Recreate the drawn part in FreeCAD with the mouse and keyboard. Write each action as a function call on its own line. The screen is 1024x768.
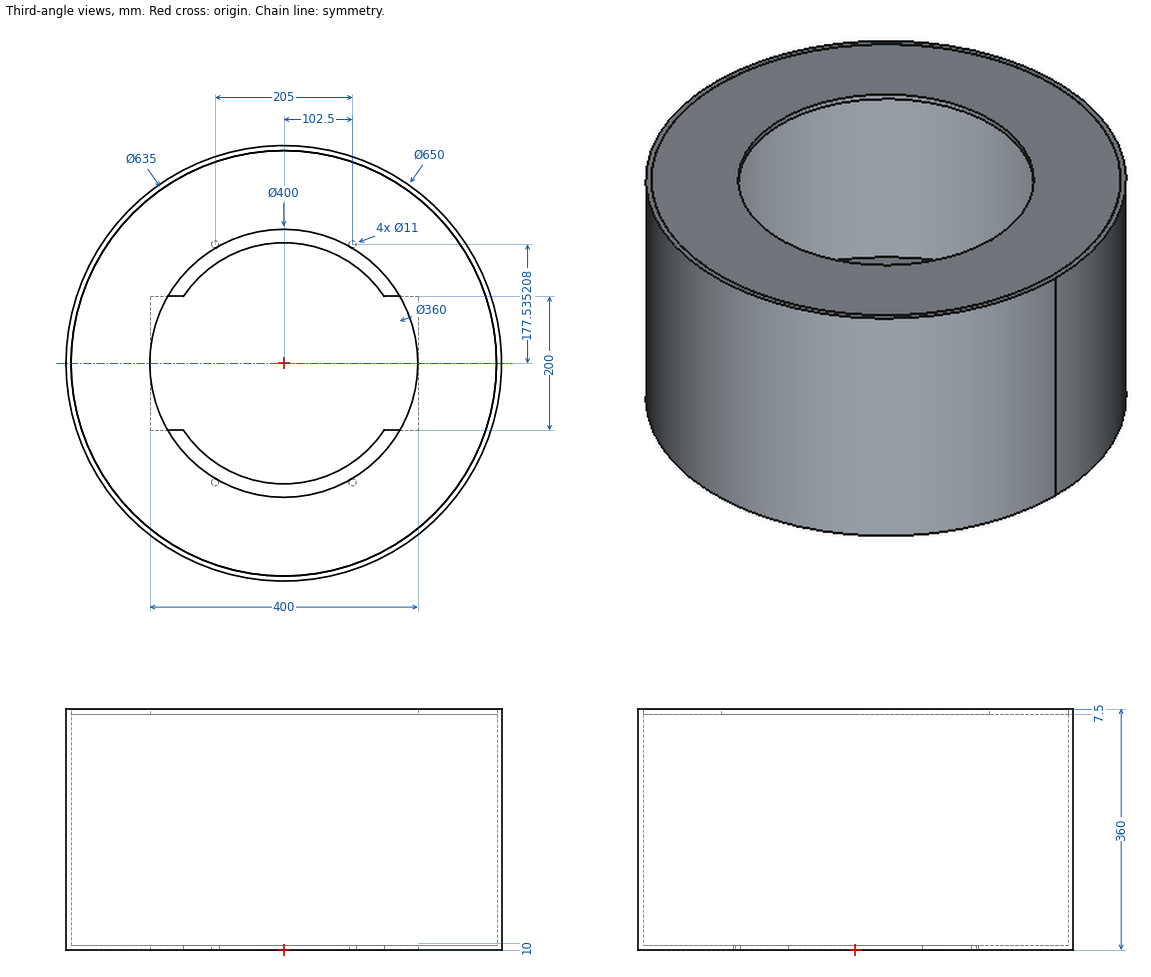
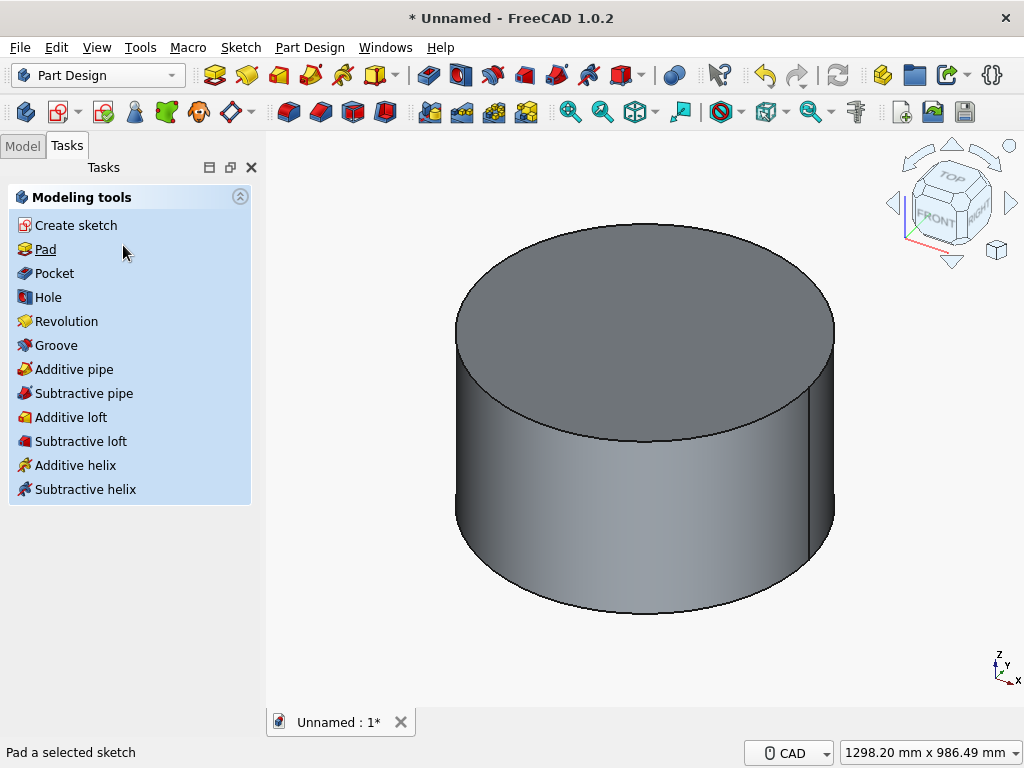
click(430, 76)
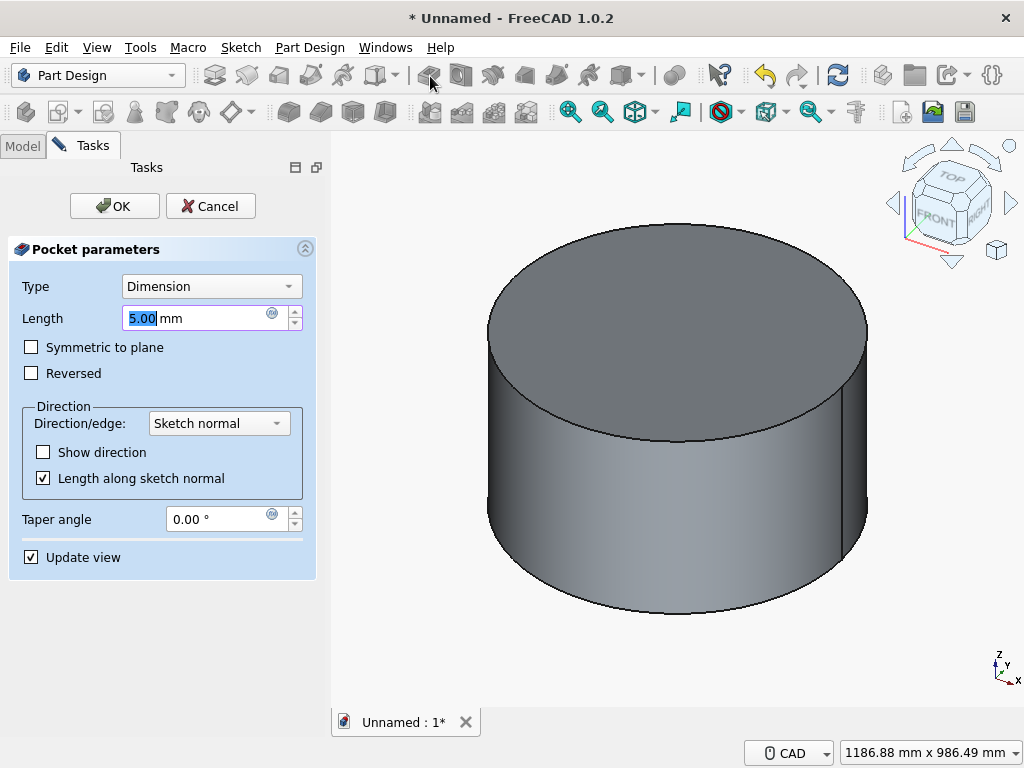
click(212, 286)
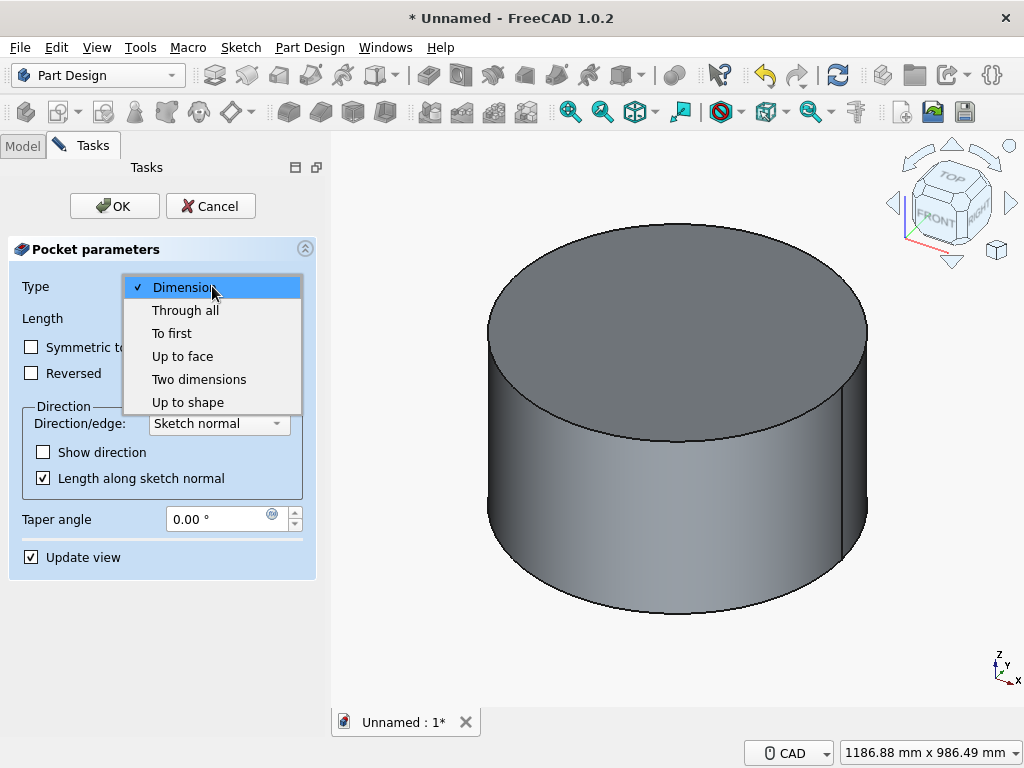
click(212, 310)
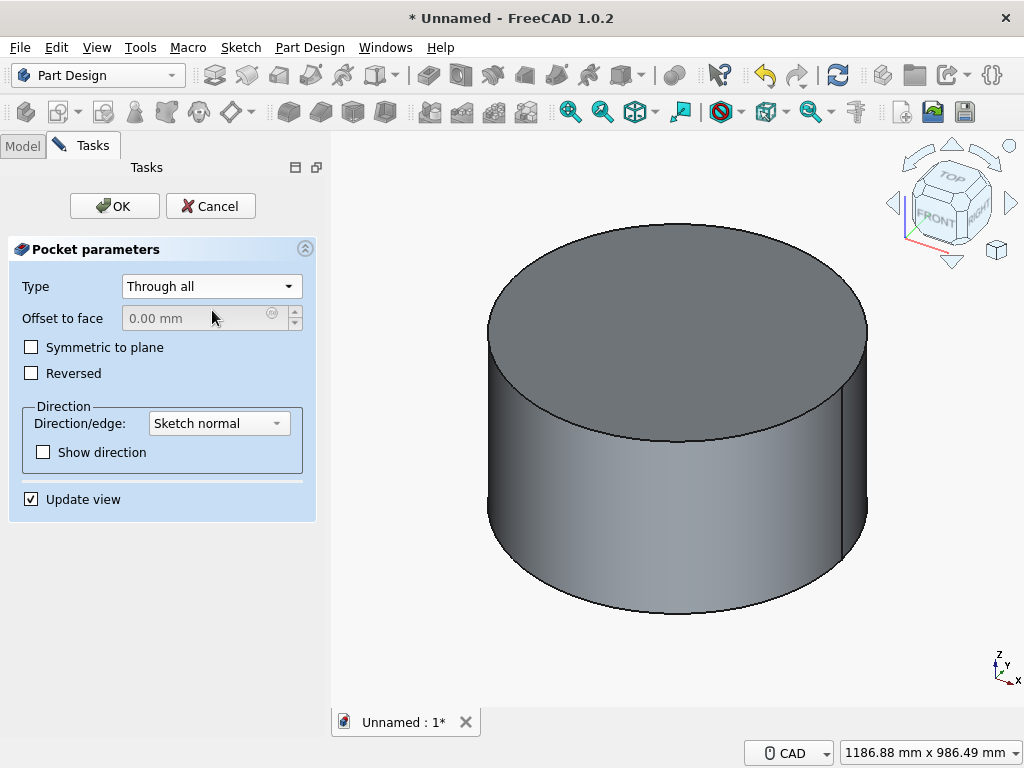
click(30, 373)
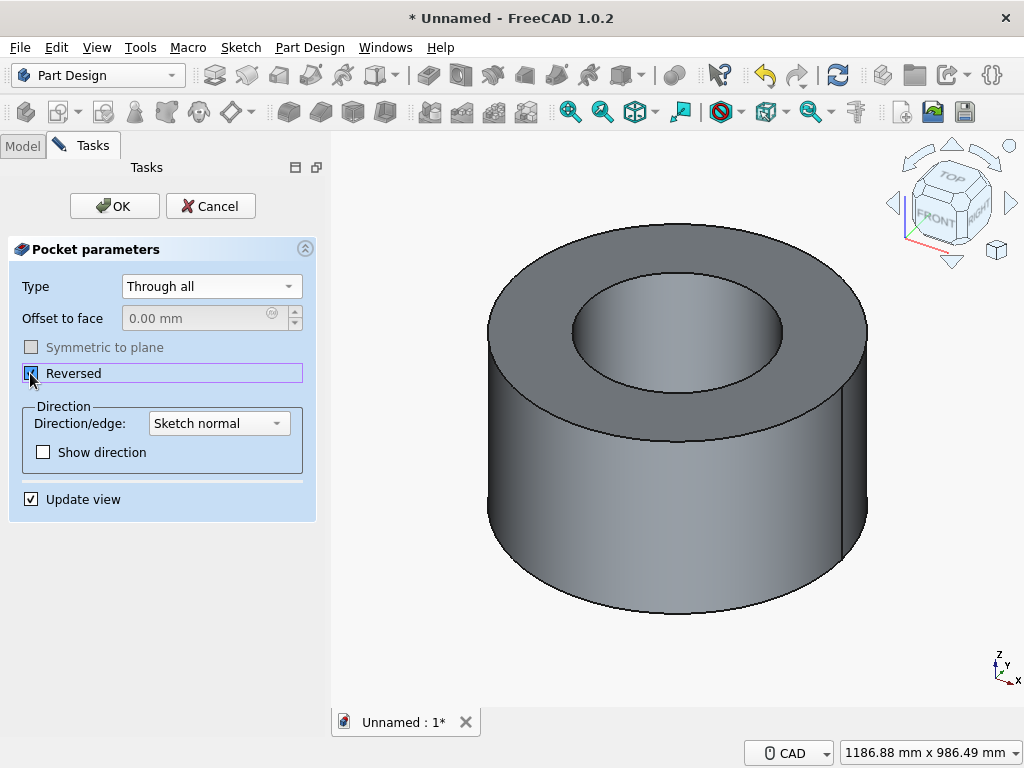
click(115, 206)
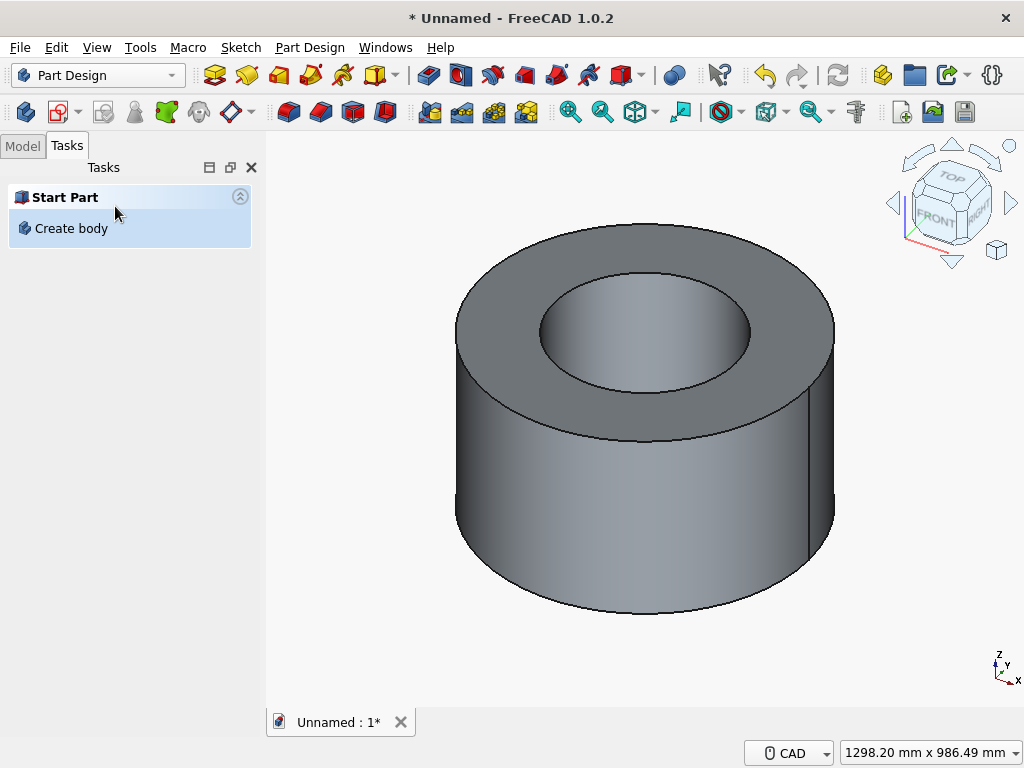
click(23, 145)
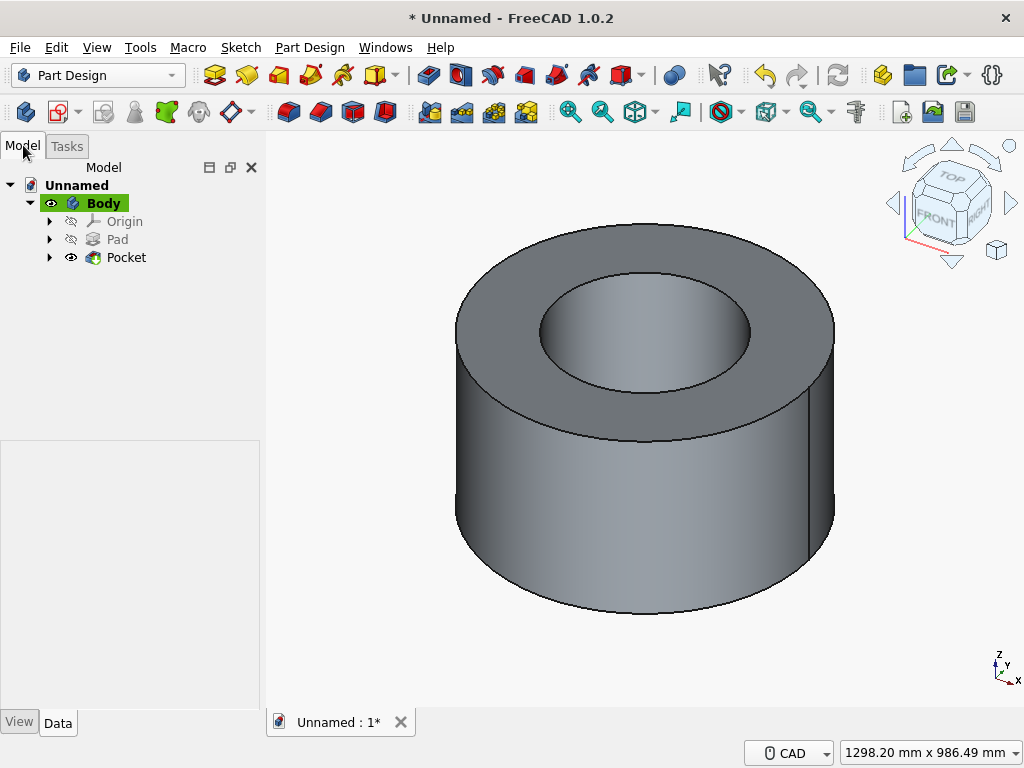
click(50, 221)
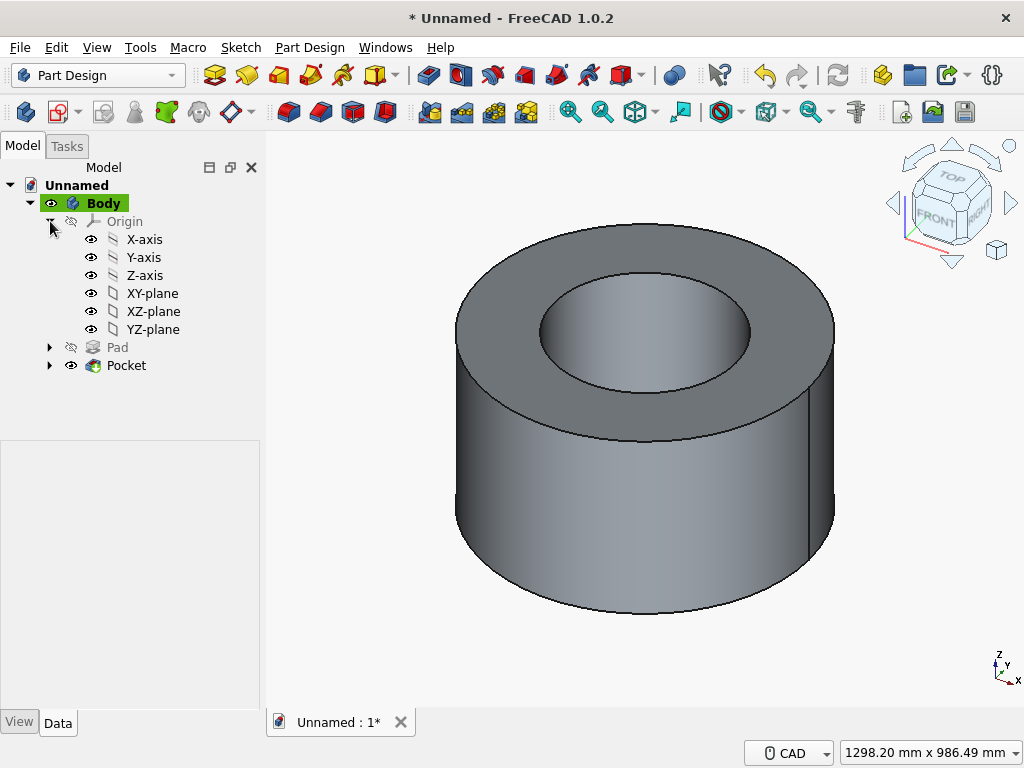
click(136, 293)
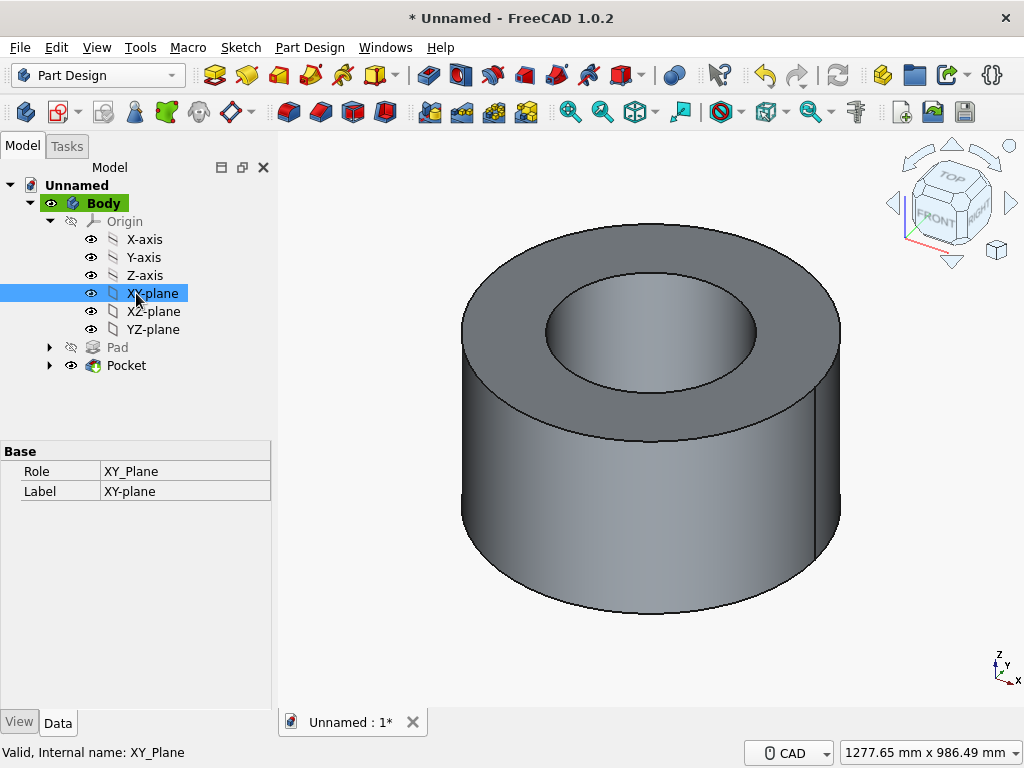
click(232, 112)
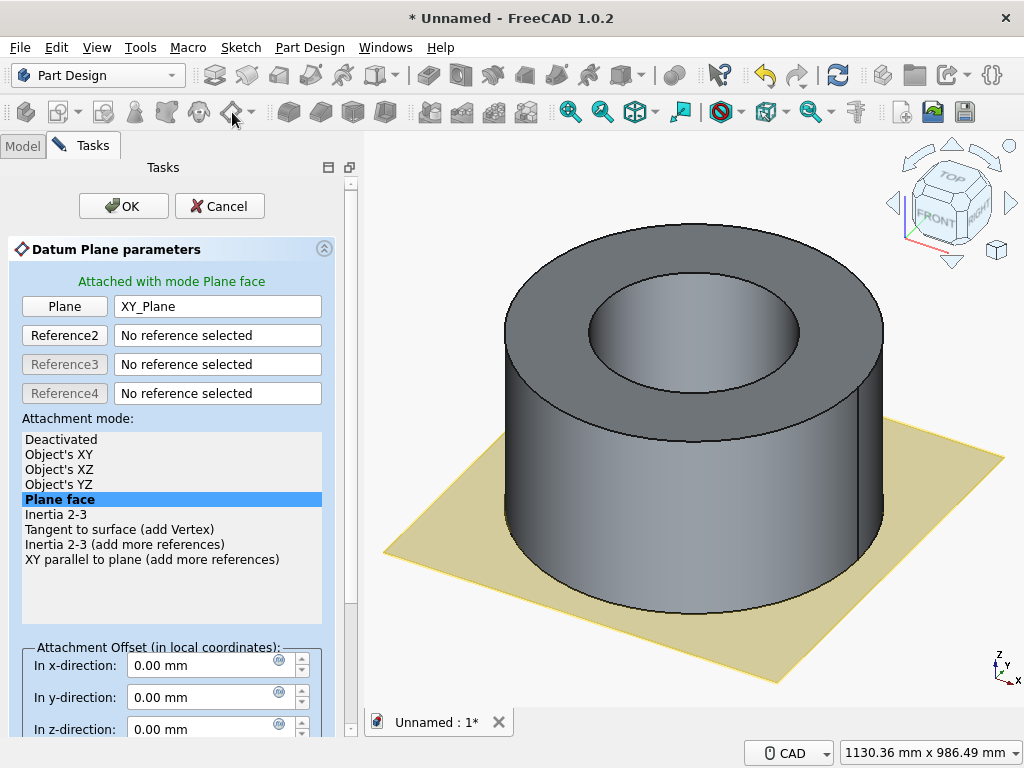
scroll(351, 456, down, 2)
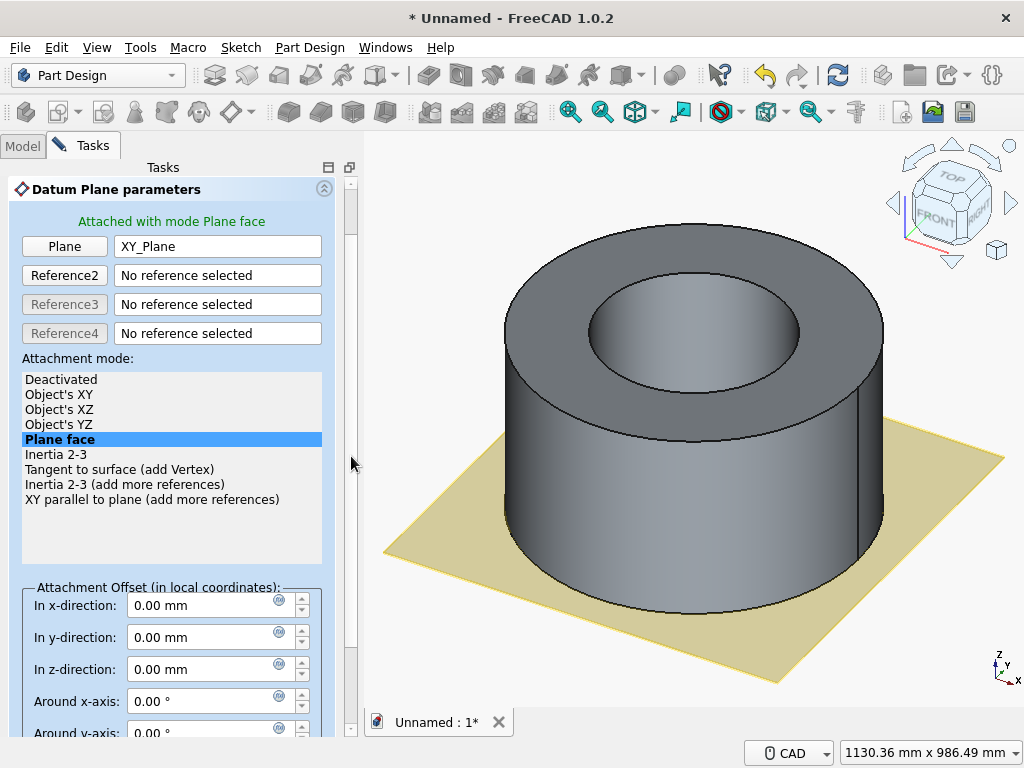
triple_click(210, 609)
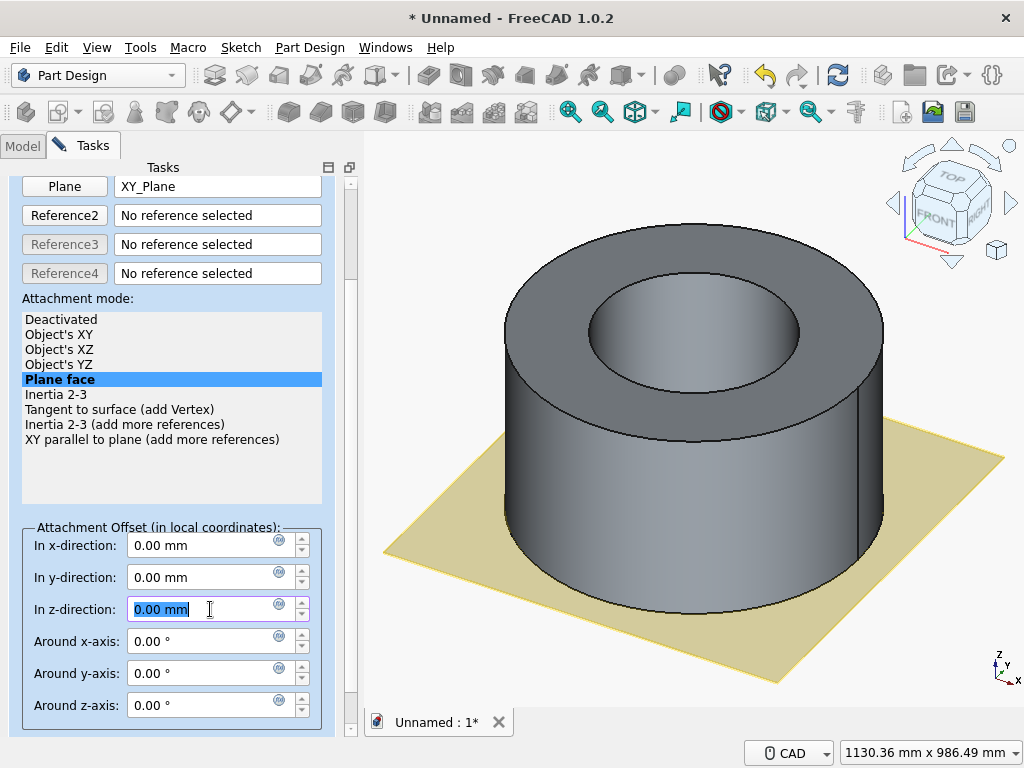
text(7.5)
key(Tab)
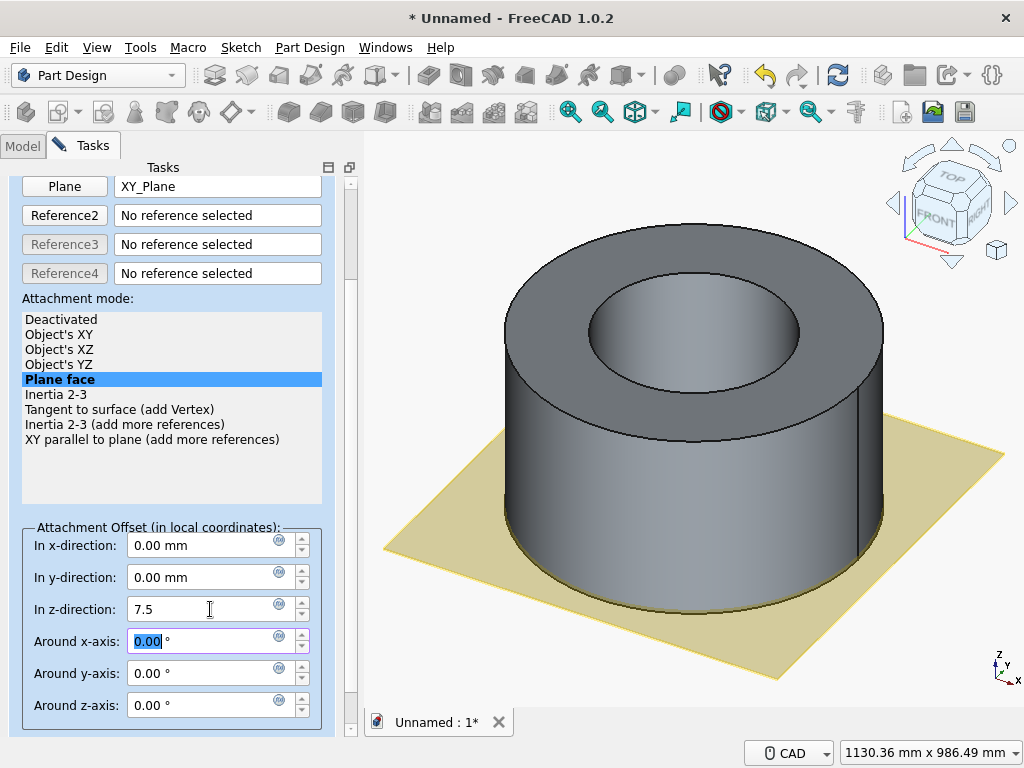
scroll(351, 456, up, 3)